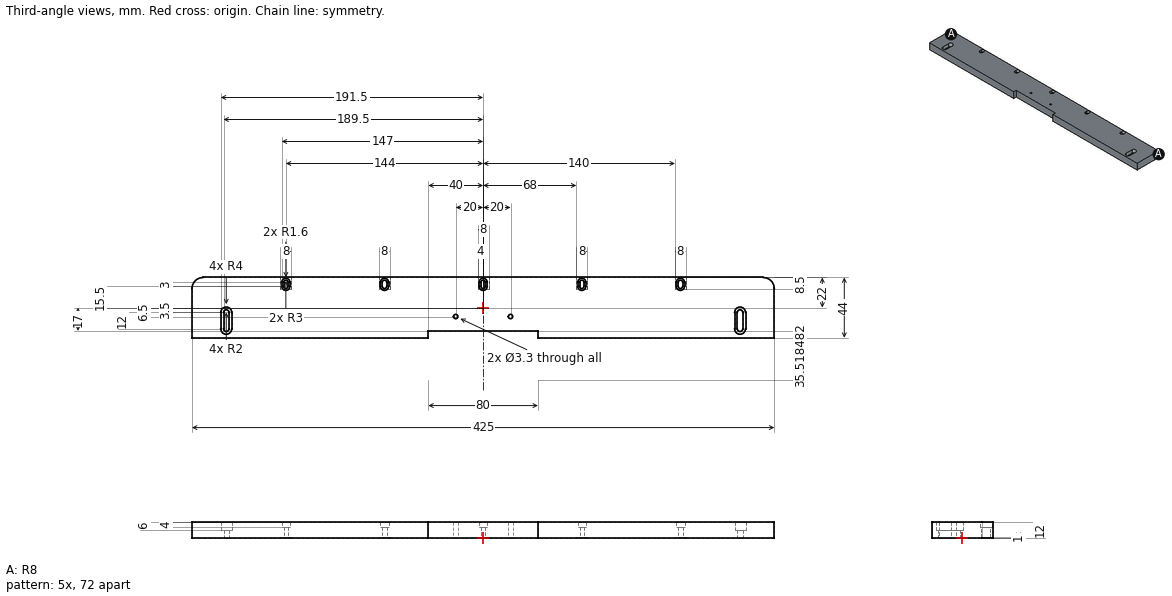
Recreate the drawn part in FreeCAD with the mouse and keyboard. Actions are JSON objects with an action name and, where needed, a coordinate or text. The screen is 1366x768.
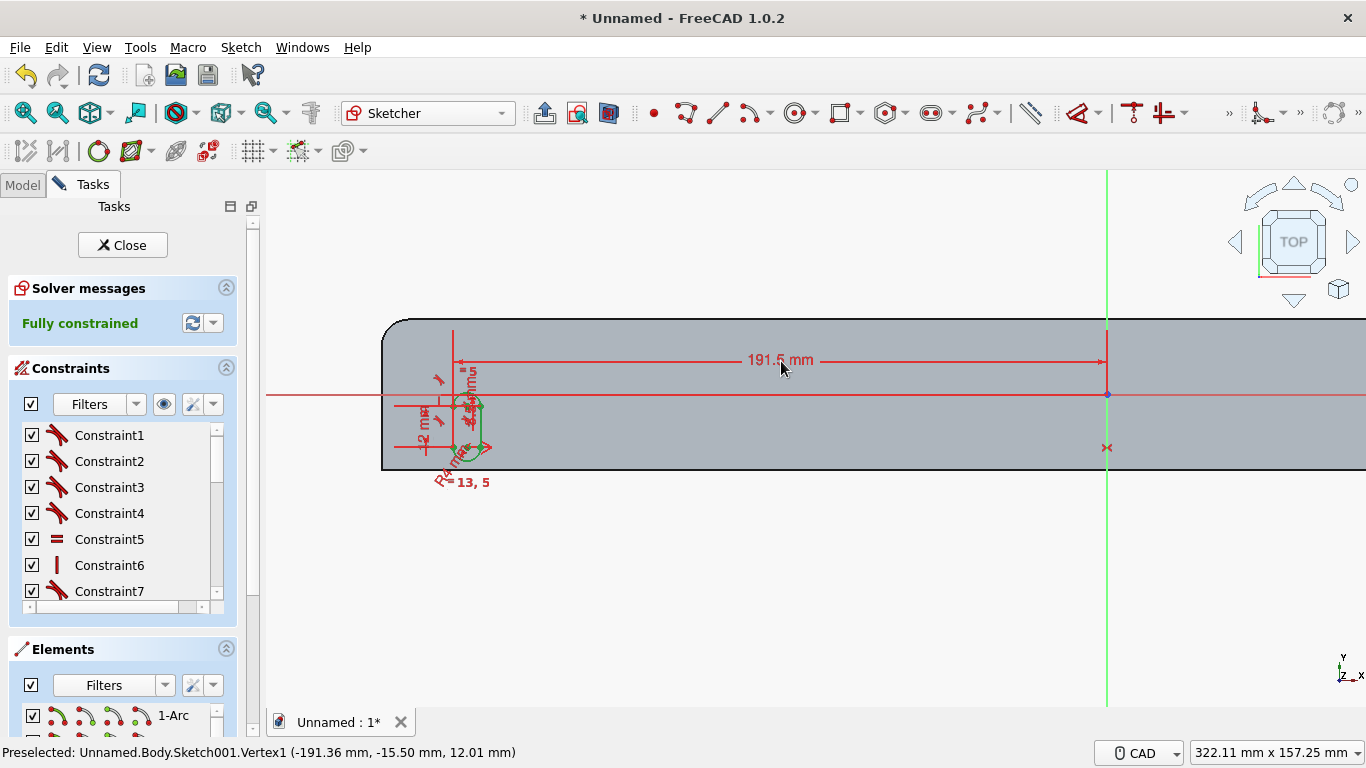
{"action": "left_click", "coordinate": [123, 245]}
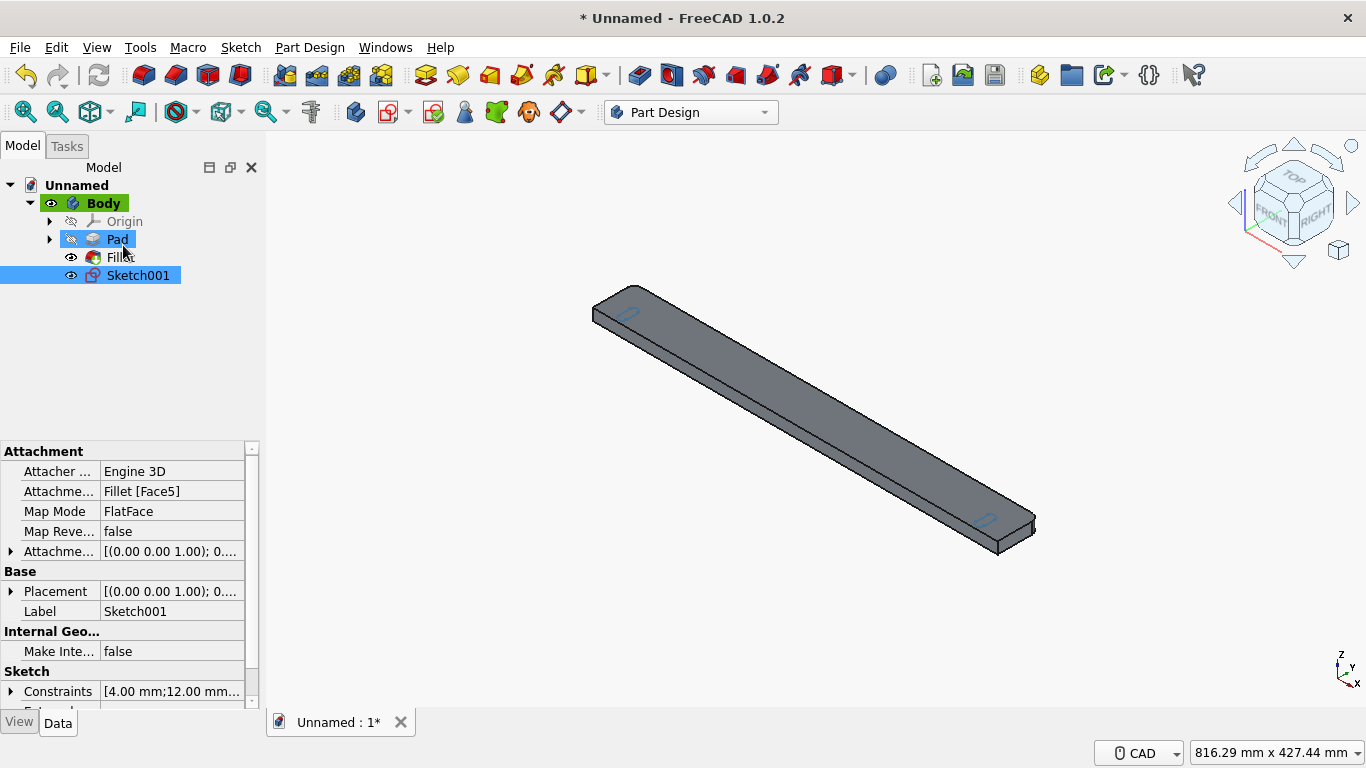
{"action": "left_click", "coordinate": [640, 76]}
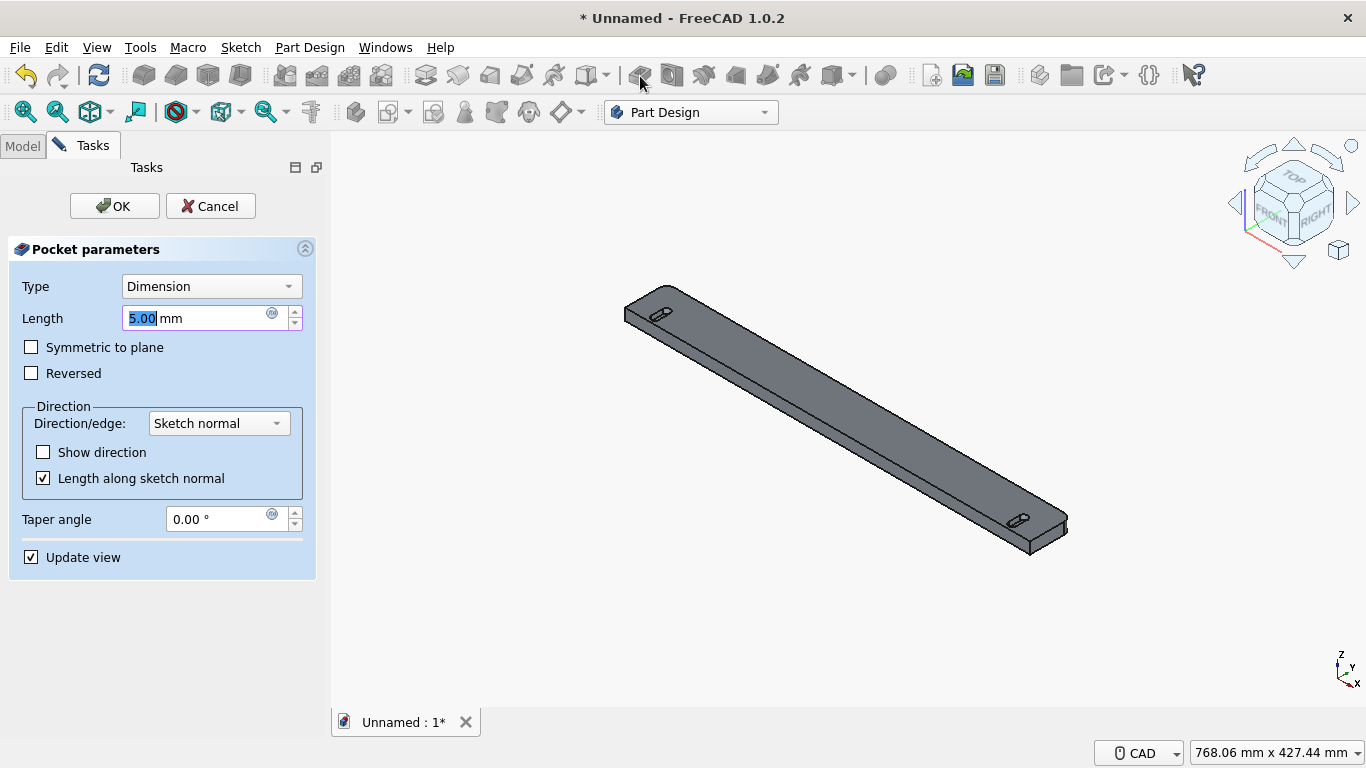
{"action": "type", "text": "6"}
{"action": "key", "text": "Tab"}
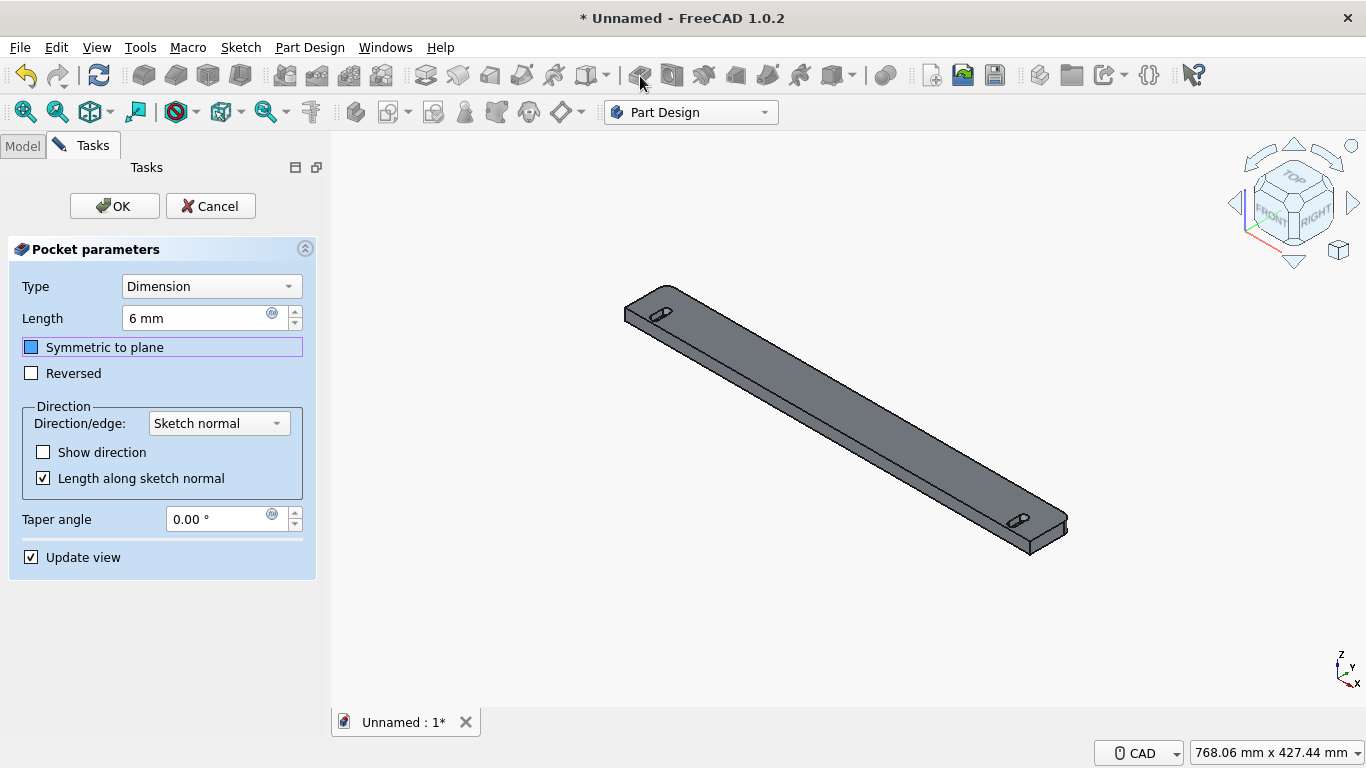
{"action": "left_click", "coordinate": [115, 206]}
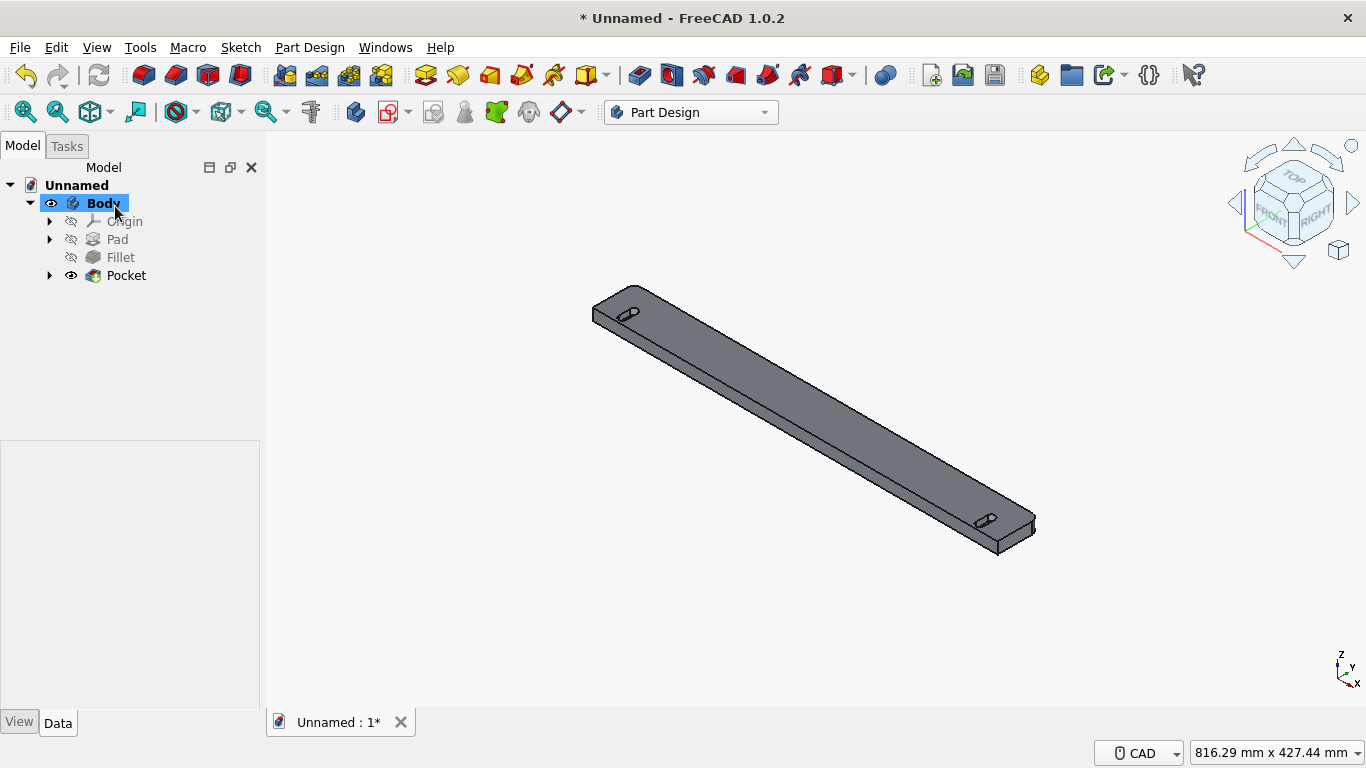
{"action": "scroll", "coordinate": [991, 523], "scroll_direction": "up", "scroll_amount": 5}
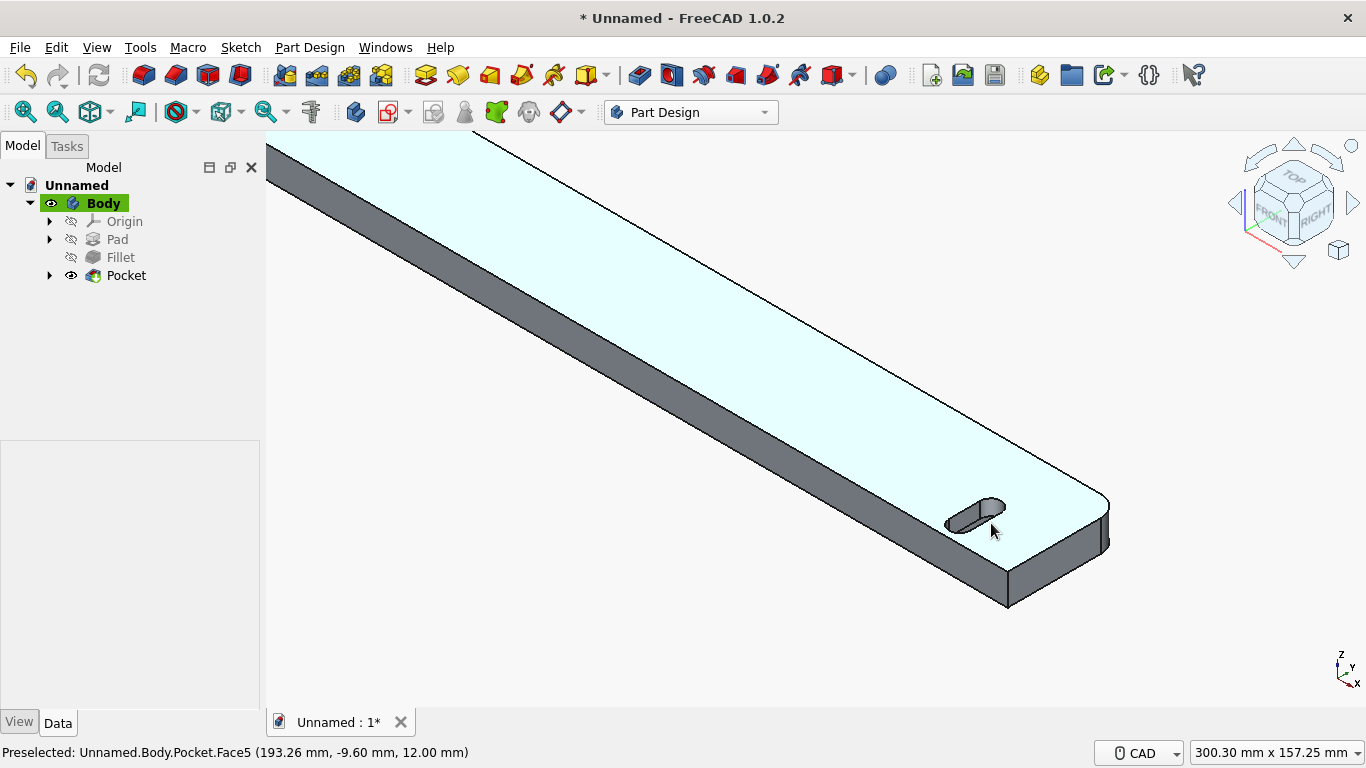
{"action": "left_click", "coordinate": [26, 112]}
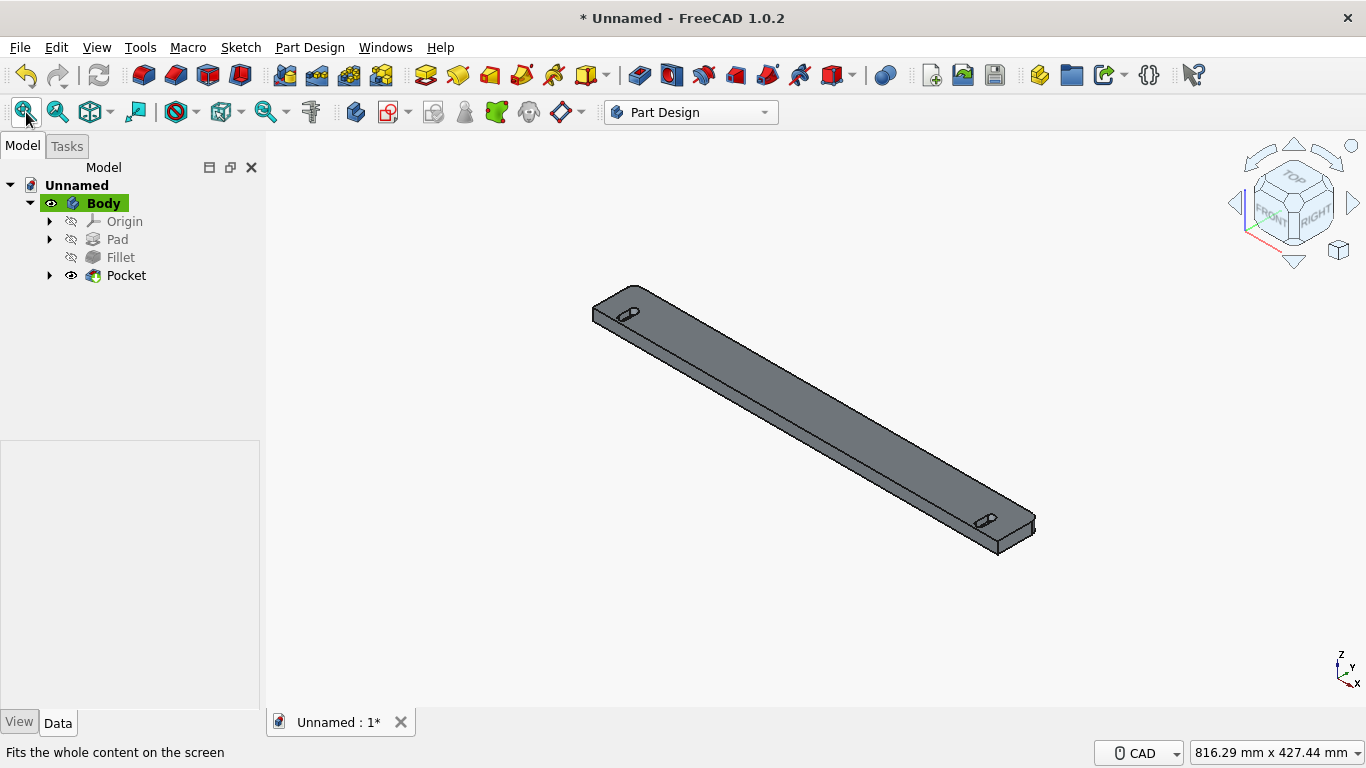
{"action": "key", "text": "2"}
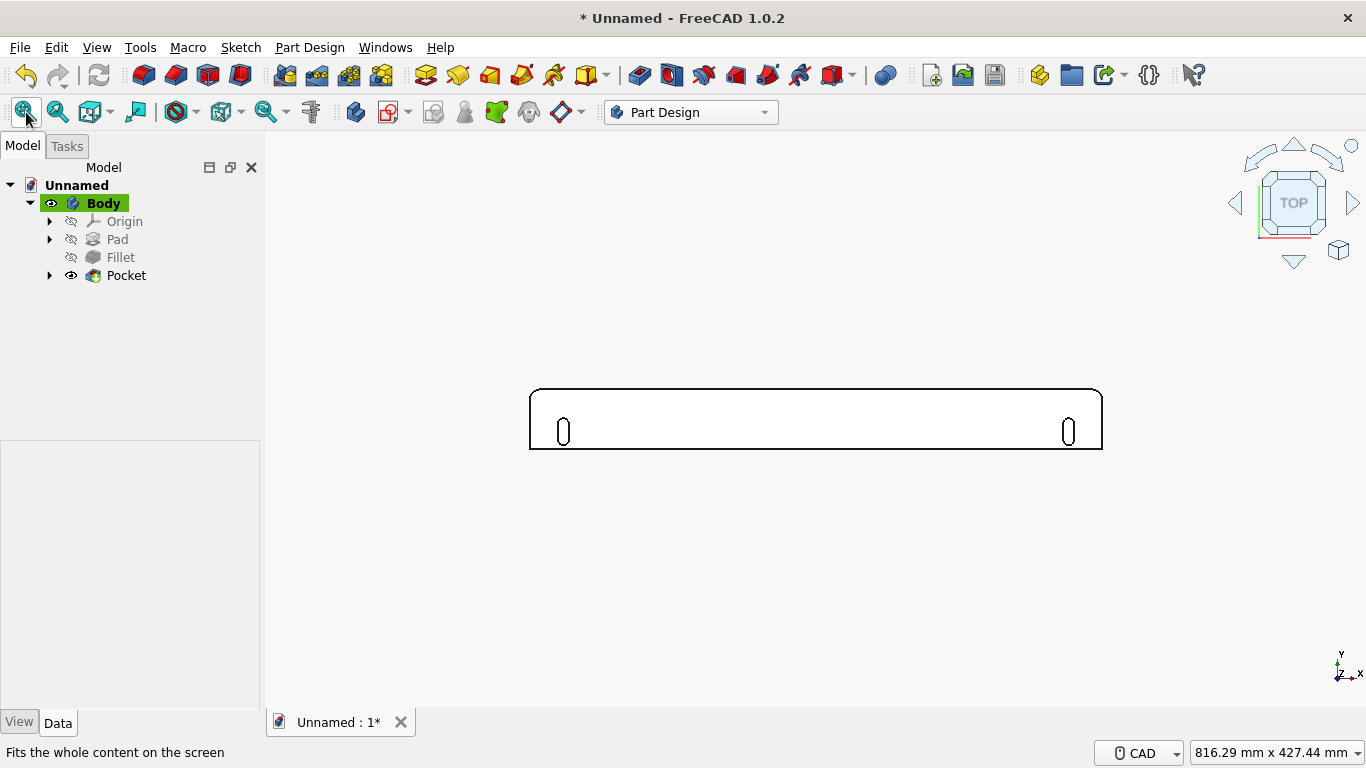
{"action": "scroll", "coordinate": [1069, 423], "scroll_direction": "up", "scroll_amount": 5}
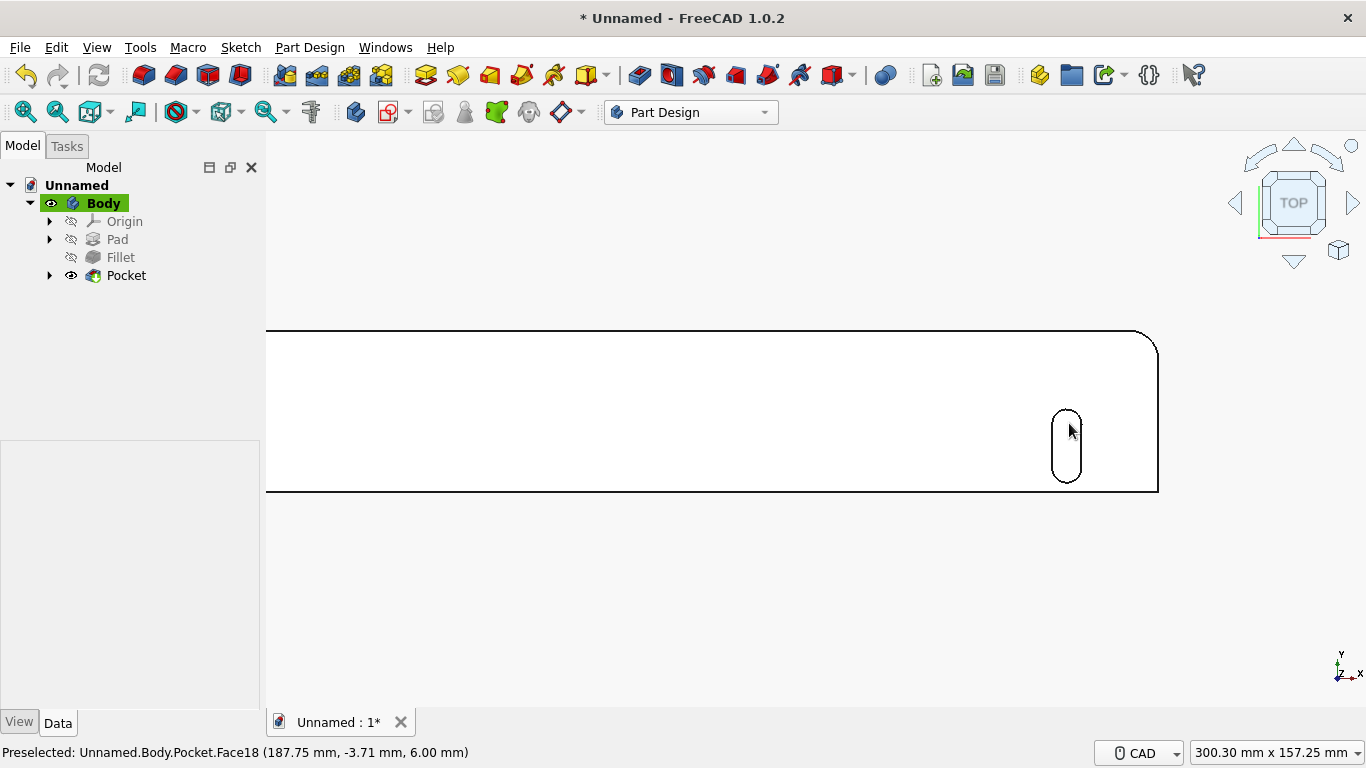
{"action": "left_click", "coordinate": [1067, 424]}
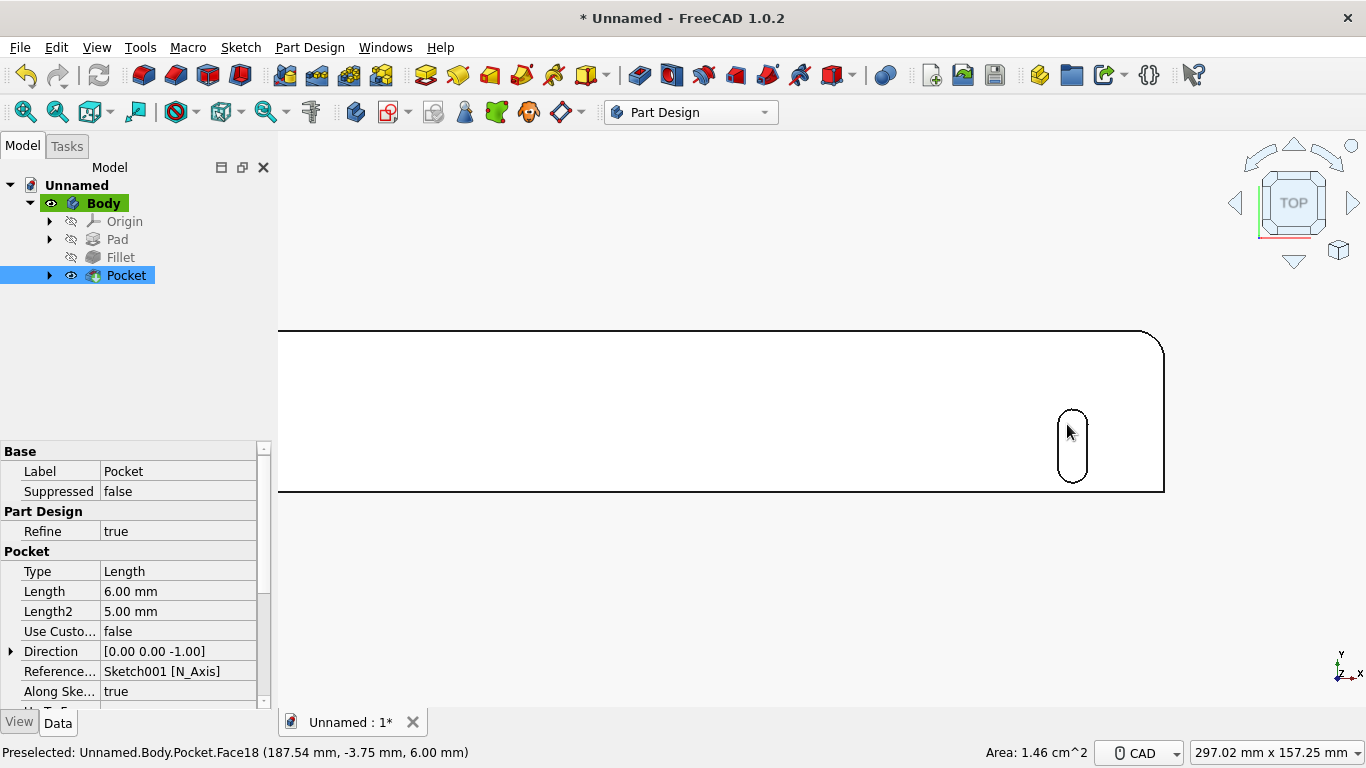
{"action": "left_click", "coordinate": [388, 112]}